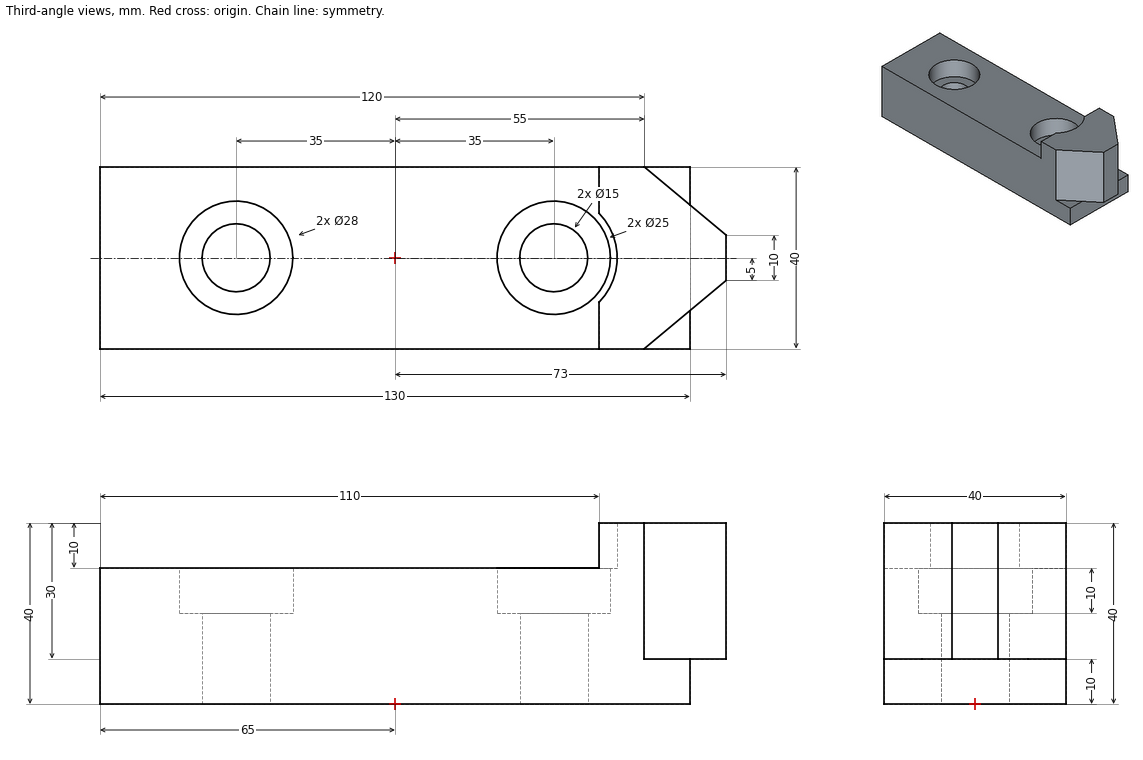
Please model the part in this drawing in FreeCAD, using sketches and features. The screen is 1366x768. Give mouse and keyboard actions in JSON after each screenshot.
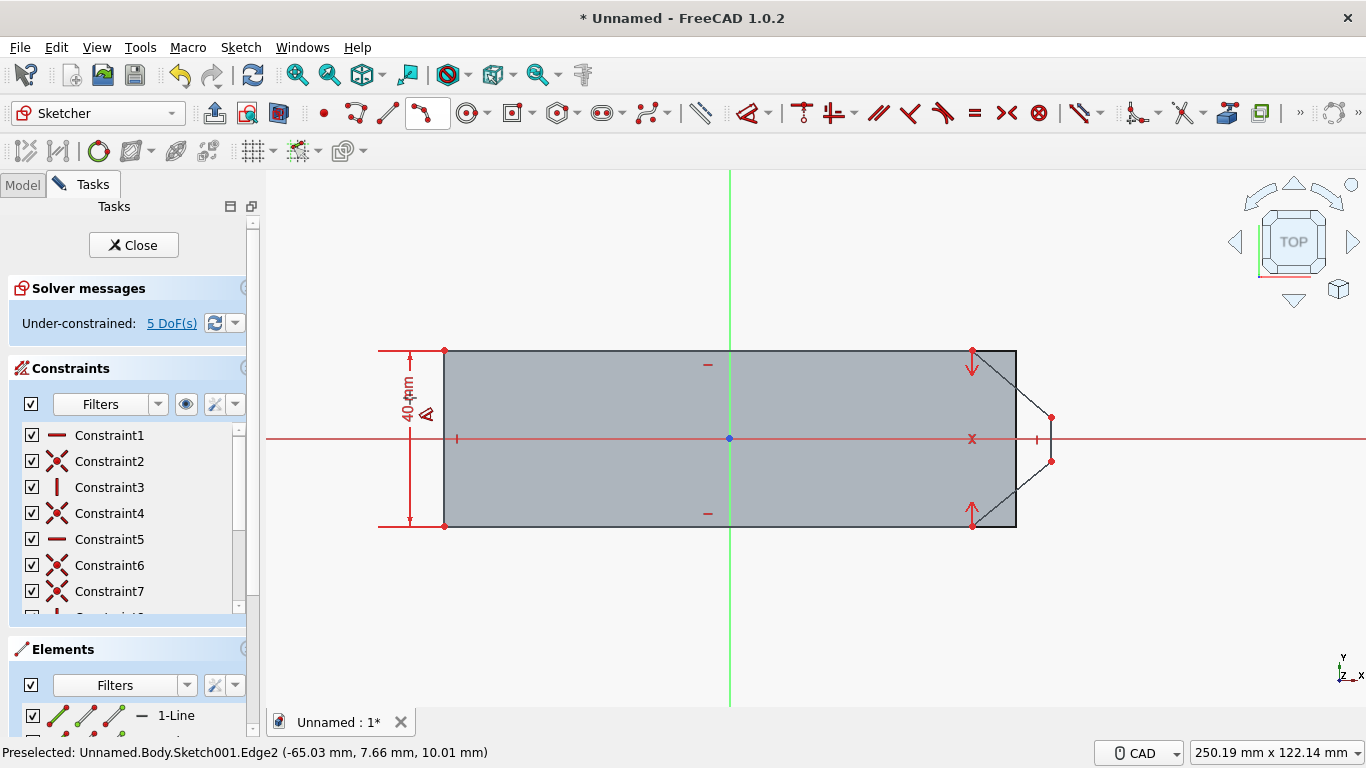
{"action": "scroll", "coordinate": [1051, 449], "scroll_direction": "up", "scroll_amount": 2}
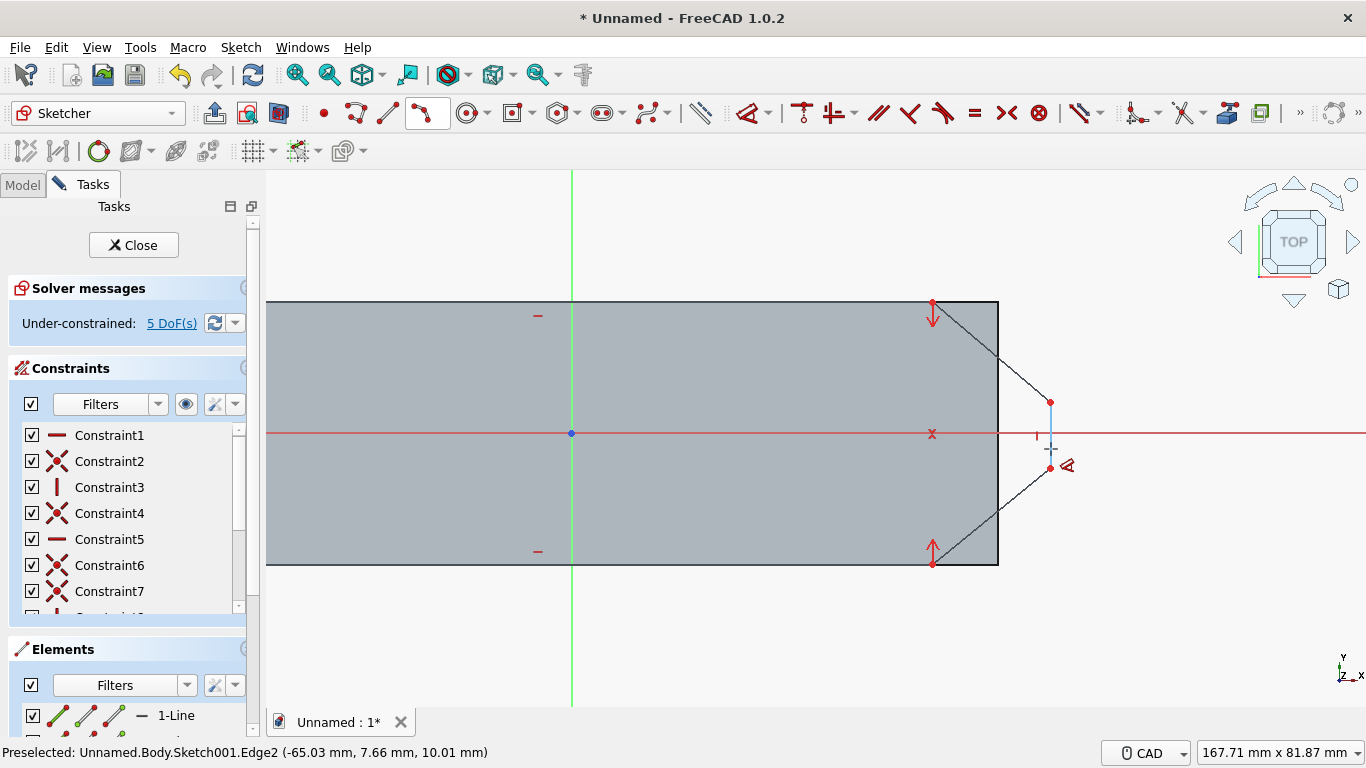
{"action": "left_click", "coordinate": [1051, 448]}
{"action": "left_click", "coordinate": [1085, 420]}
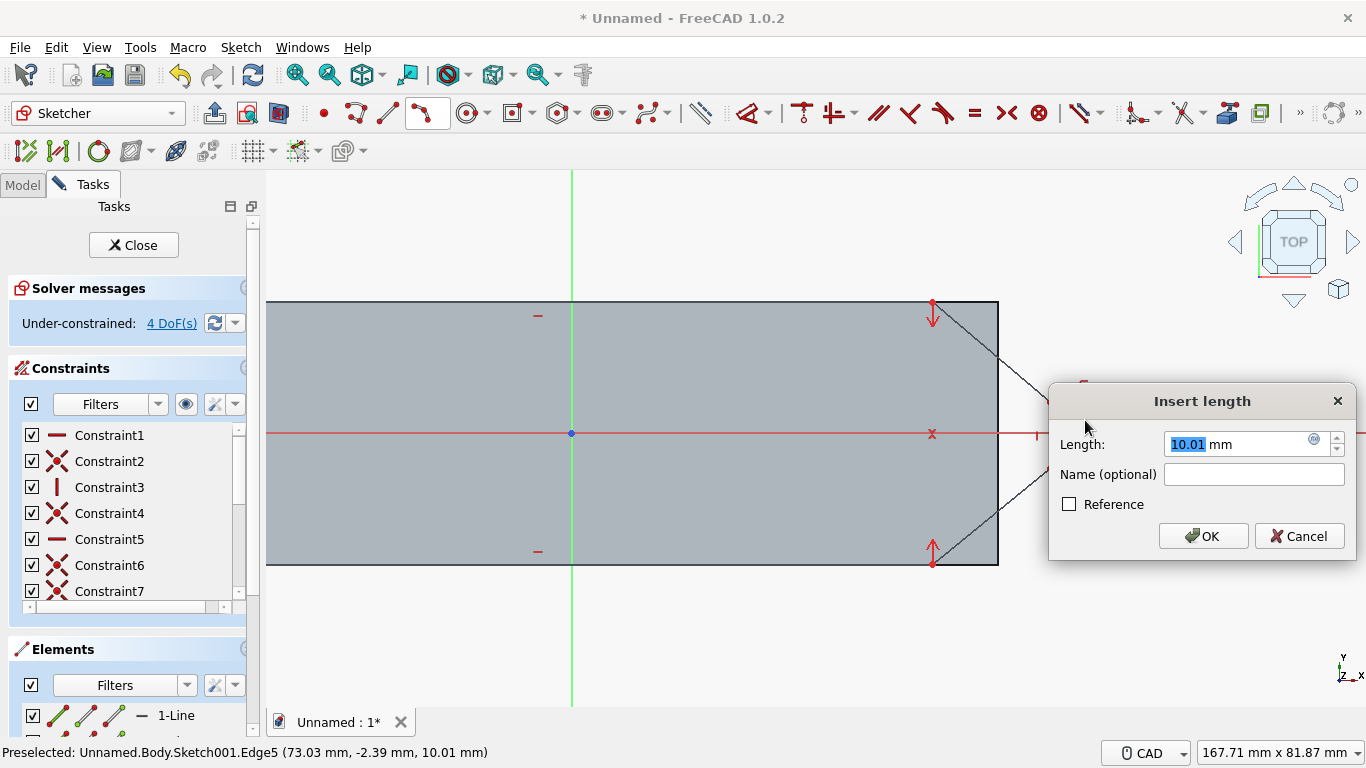
{"action": "type", "text": "10"}
{"action": "key", "text": "Return"}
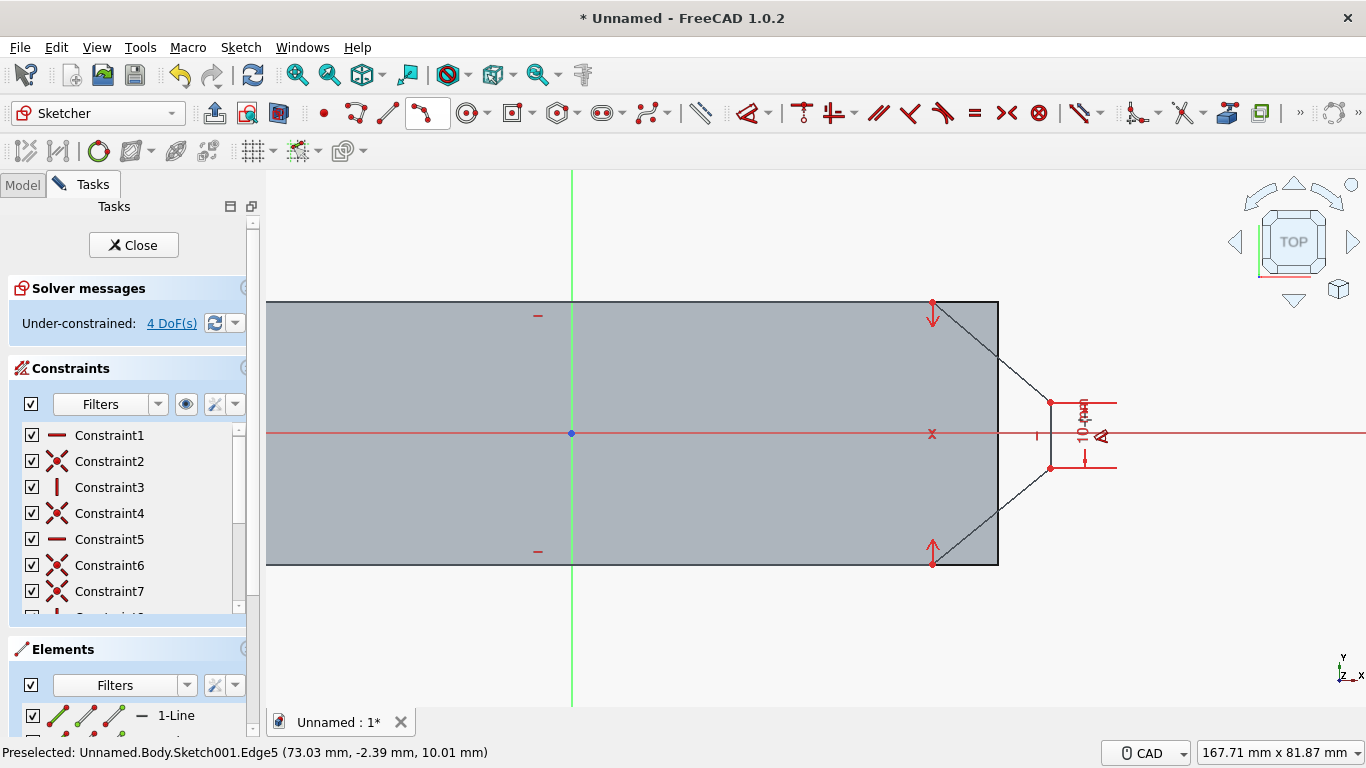
{"action": "left_click", "coordinate": [1051, 468]}
{"action": "left_click", "coordinate": [1085, 451]}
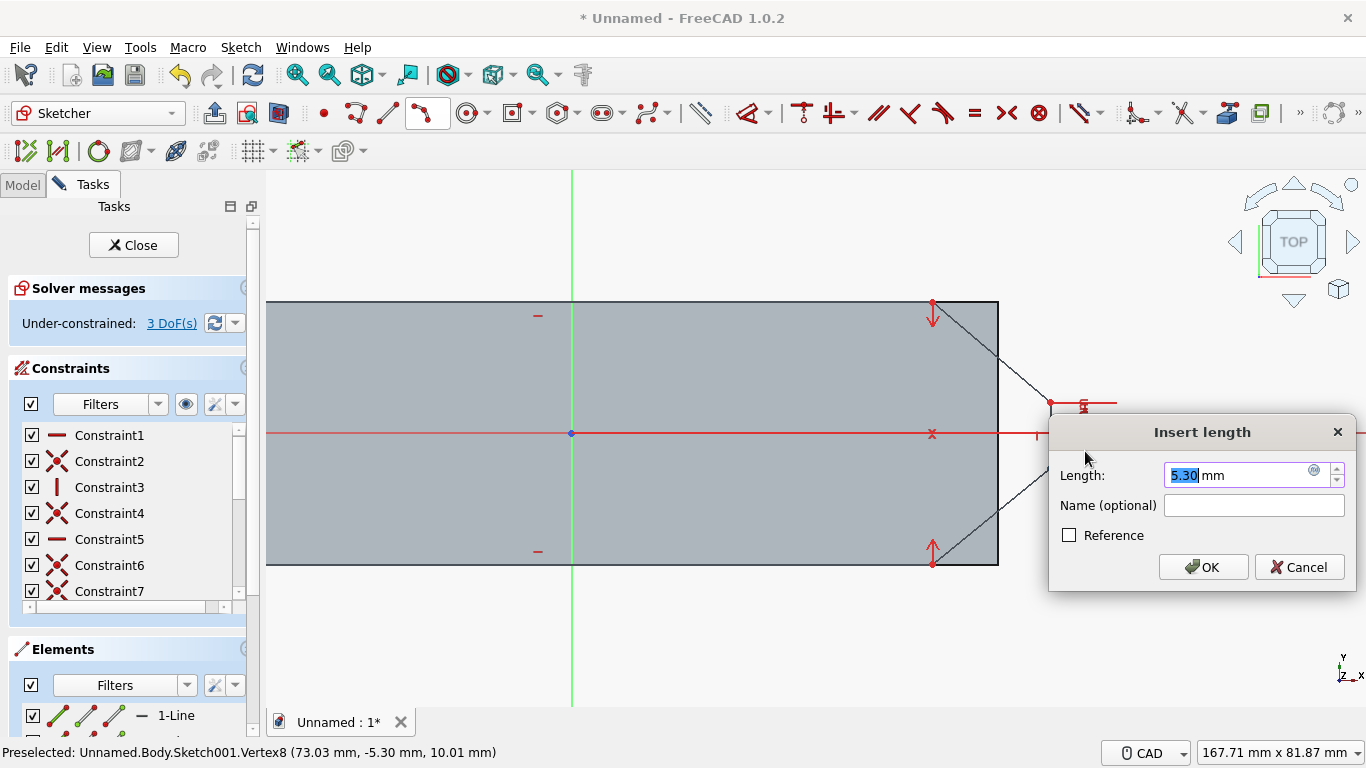
{"action": "type", "text": "5"}
{"action": "key", "text": "Return"}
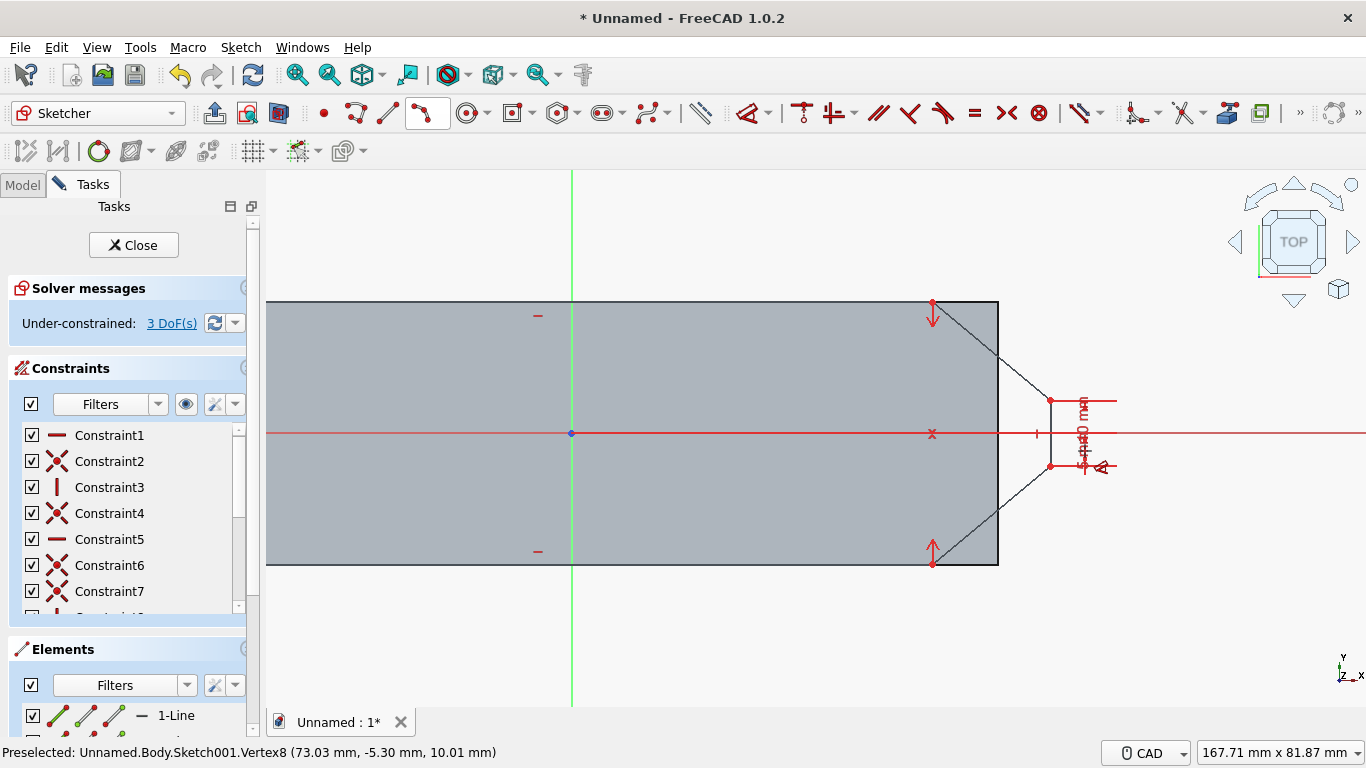
{"action": "left_click", "coordinate": [696, 302]}
{"action": "left_click", "coordinate": [613, 268]}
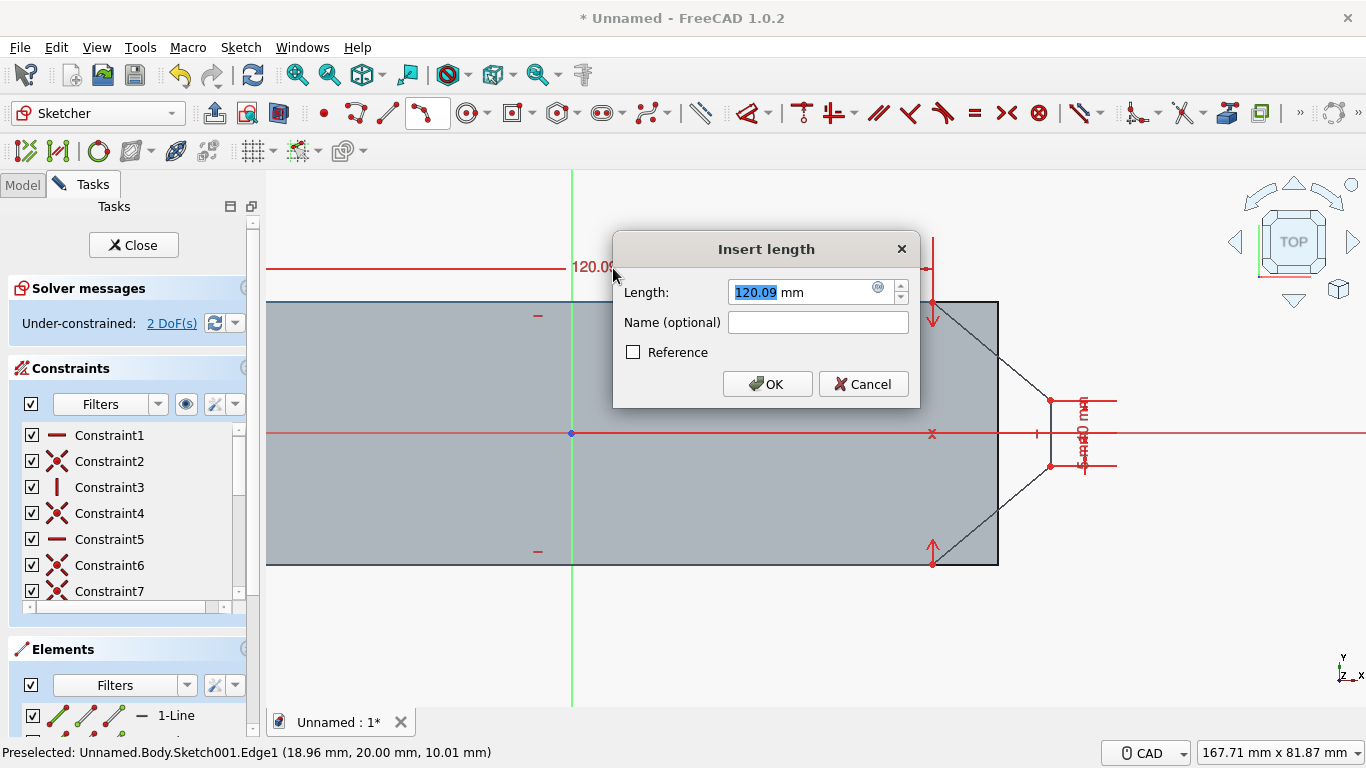
{"action": "type", "text": "120"}
{"action": "key", "text": "Return"}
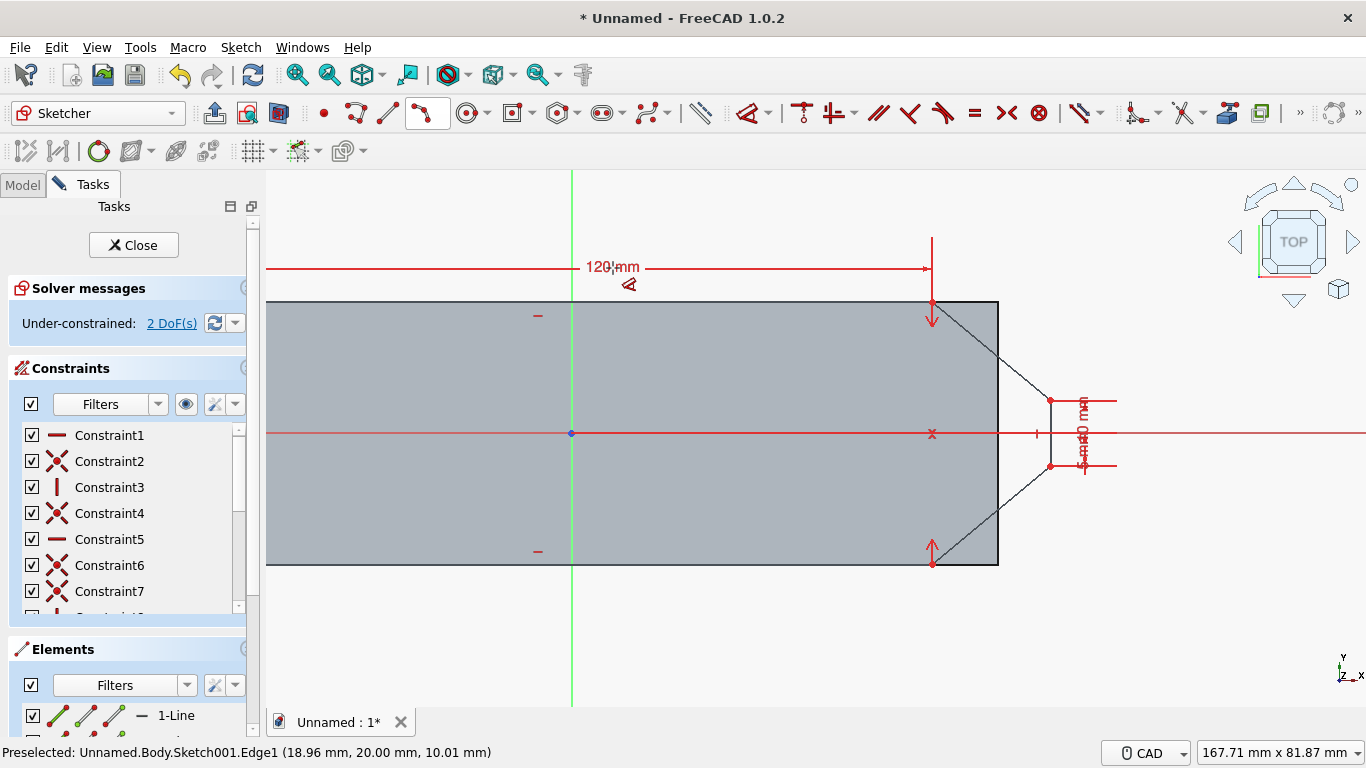
{"action": "left_click", "coordinate": [932, 302]}
{"action": "left_click", "coordinate": [752, 268]}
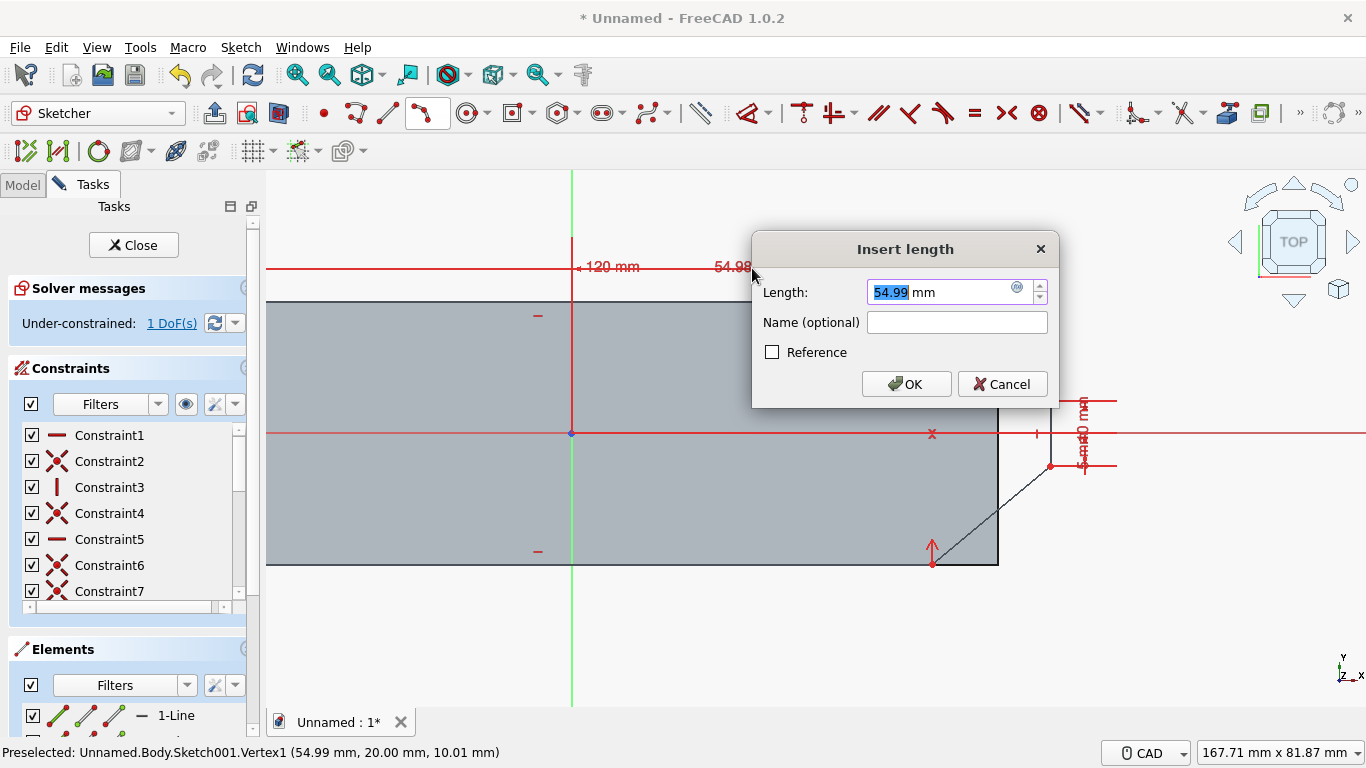
{"action": "type", "text": "55"}
{"action": "key", "text": "Return"}